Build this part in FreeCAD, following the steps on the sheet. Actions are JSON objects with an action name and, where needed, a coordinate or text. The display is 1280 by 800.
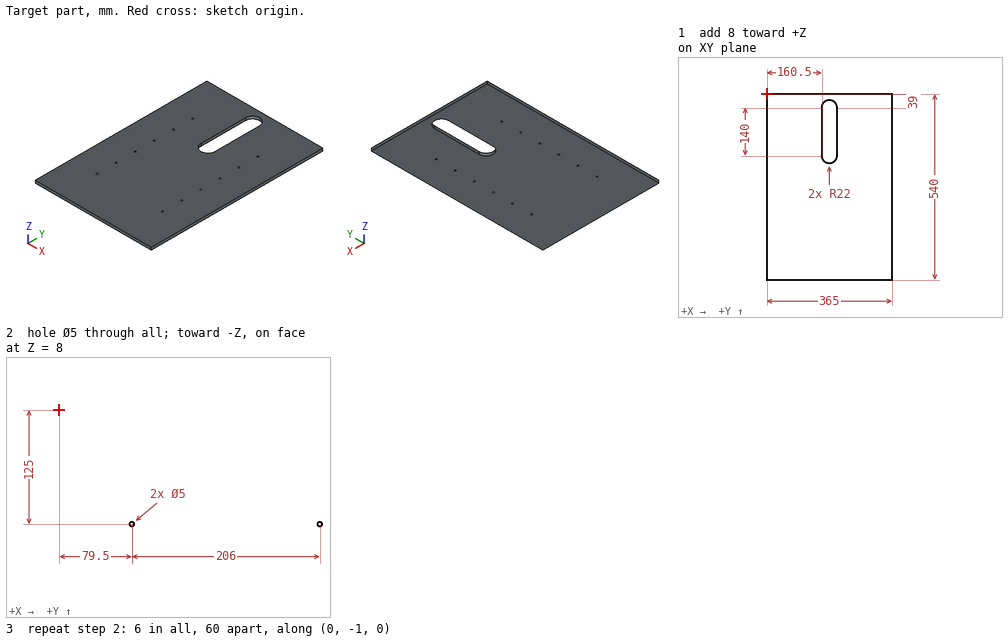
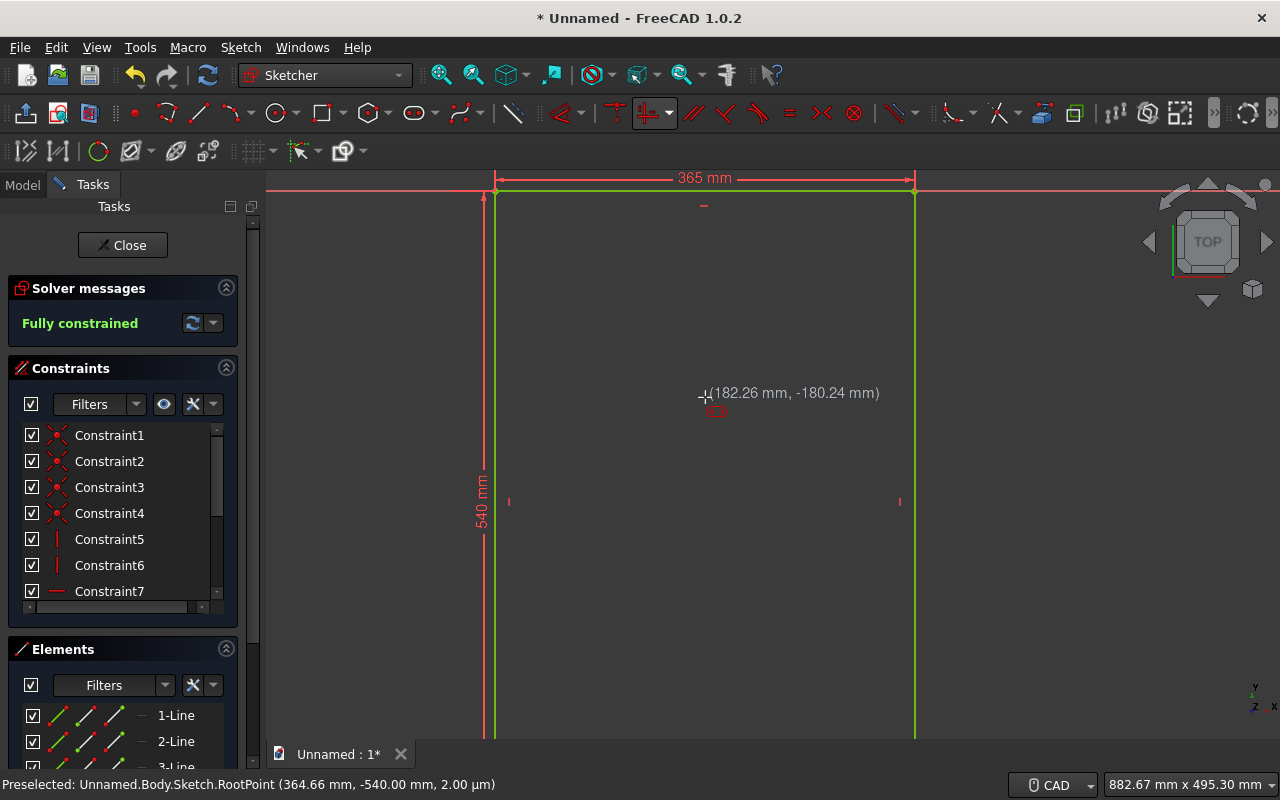
{"action": "left_click", "coordinate": [705, 397]}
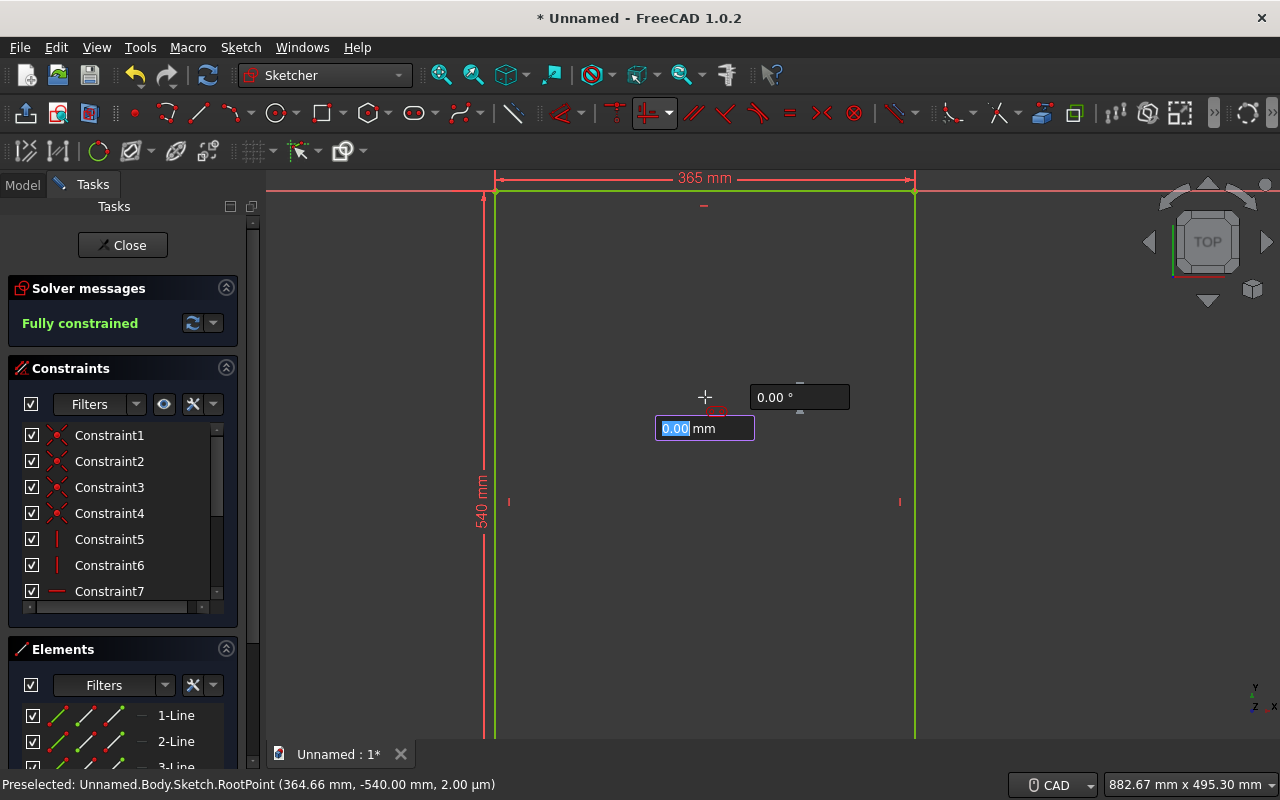
{"action": "left_click", "coordinate": [705, 236]}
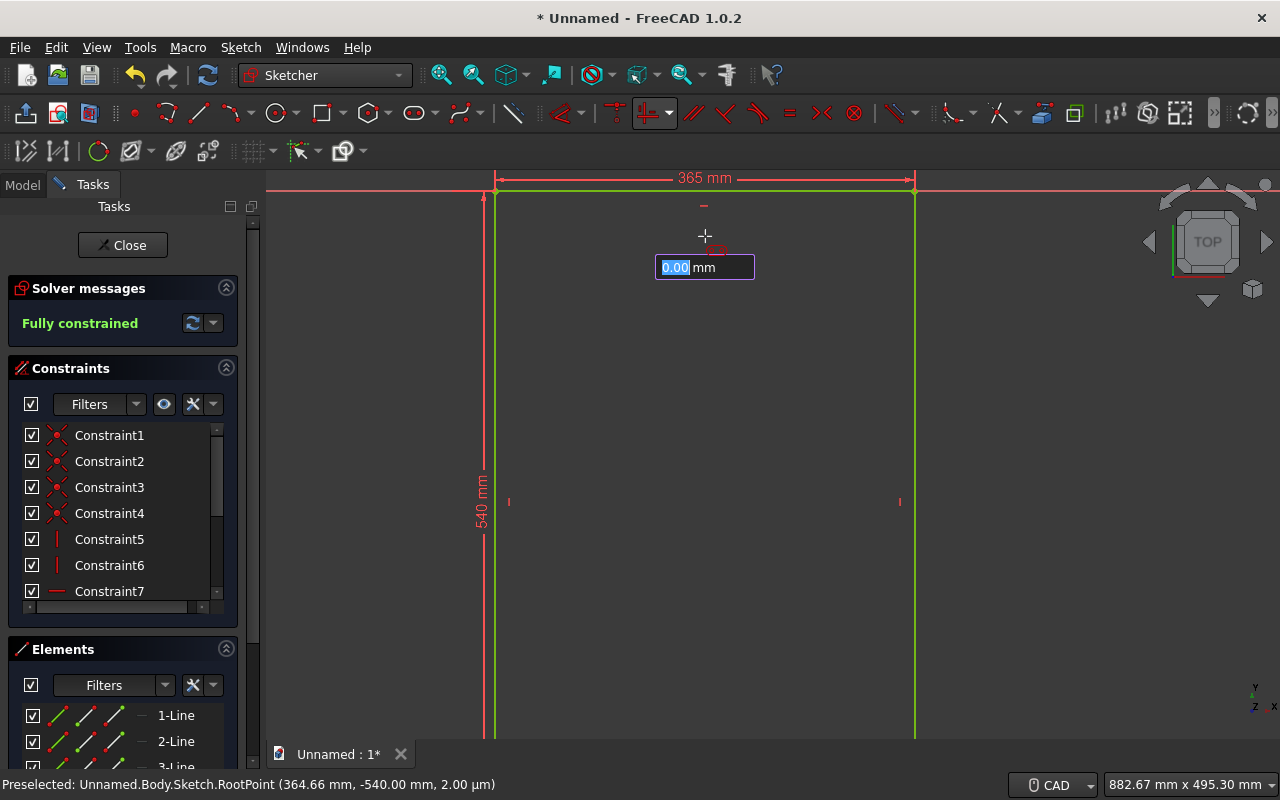
{"action": "left_click", "coordinate": [730, 317]}
{"action": "key", "text": "Escape"}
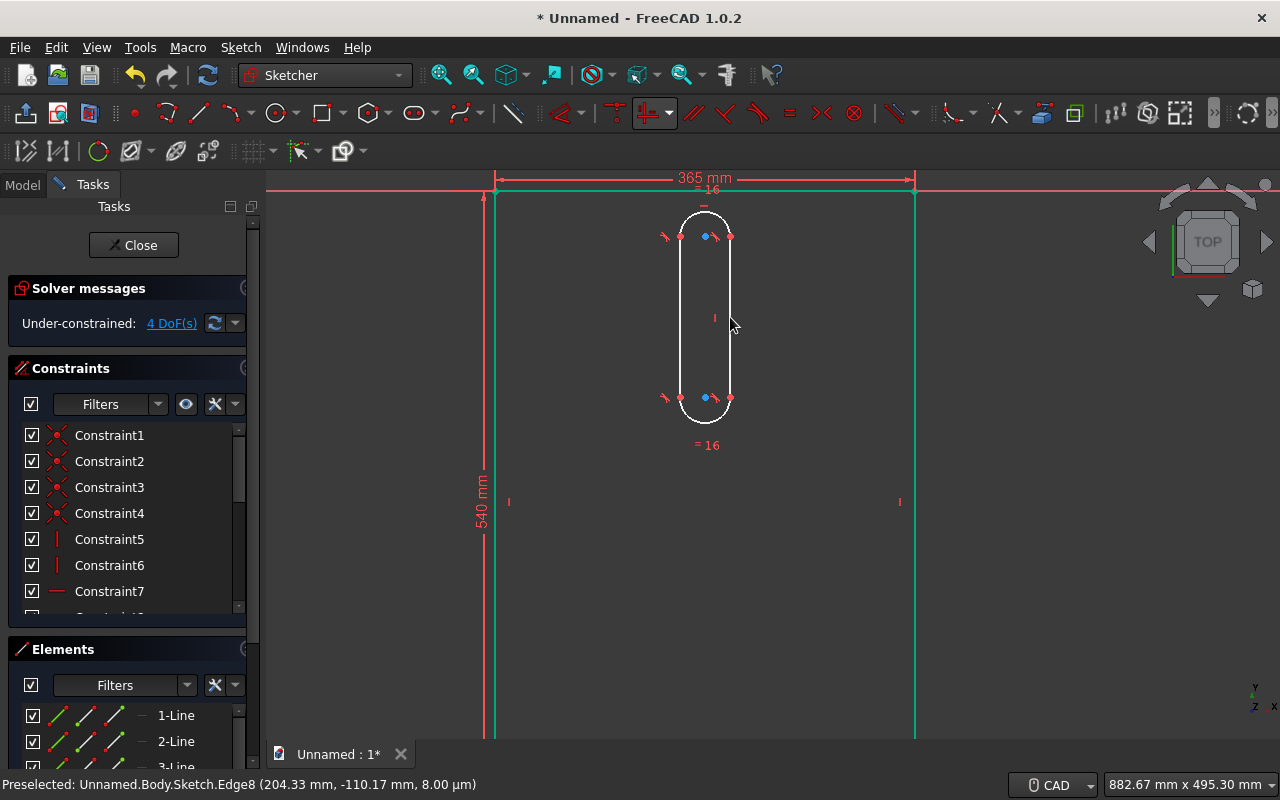
{"action": "left_click", "coordinate": [560, 114]}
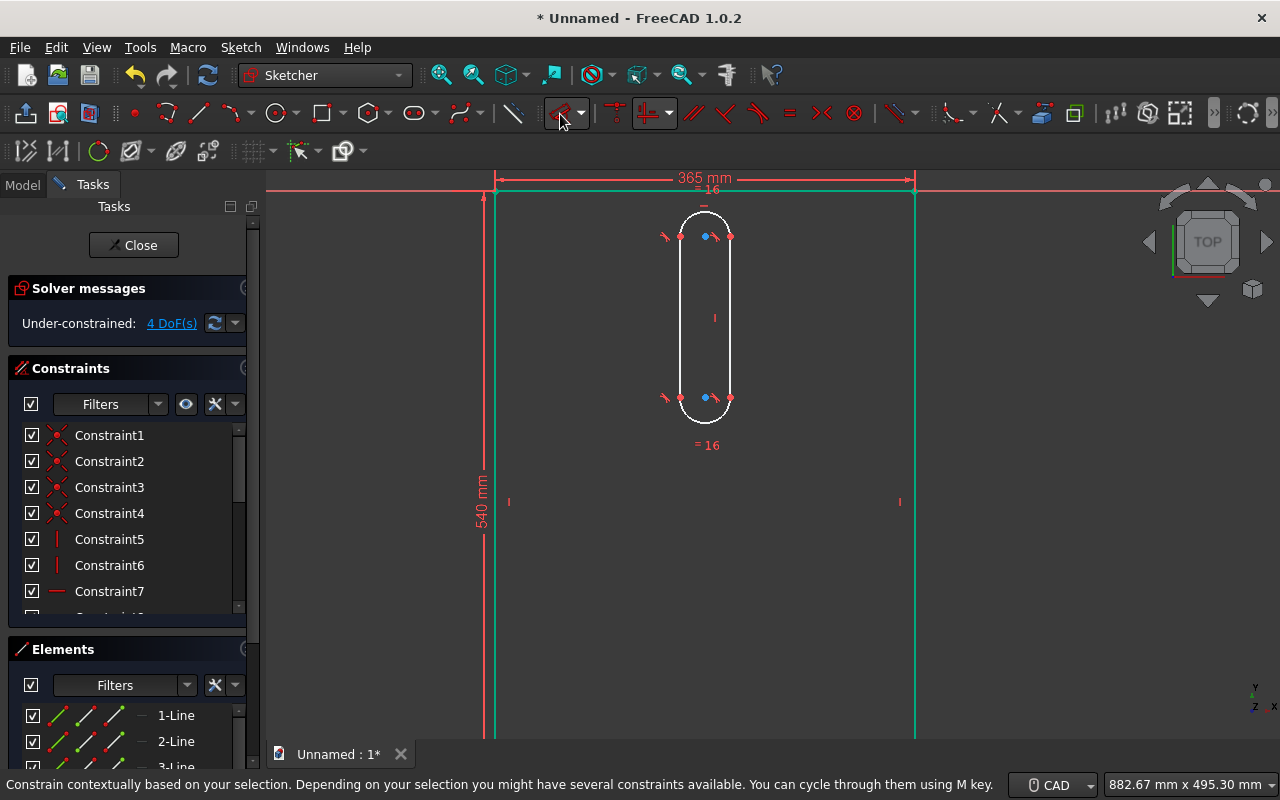
{"action": "scroll", "coordinate": [690, 418], "scroll_direction": "up", "scroll_amount": 3}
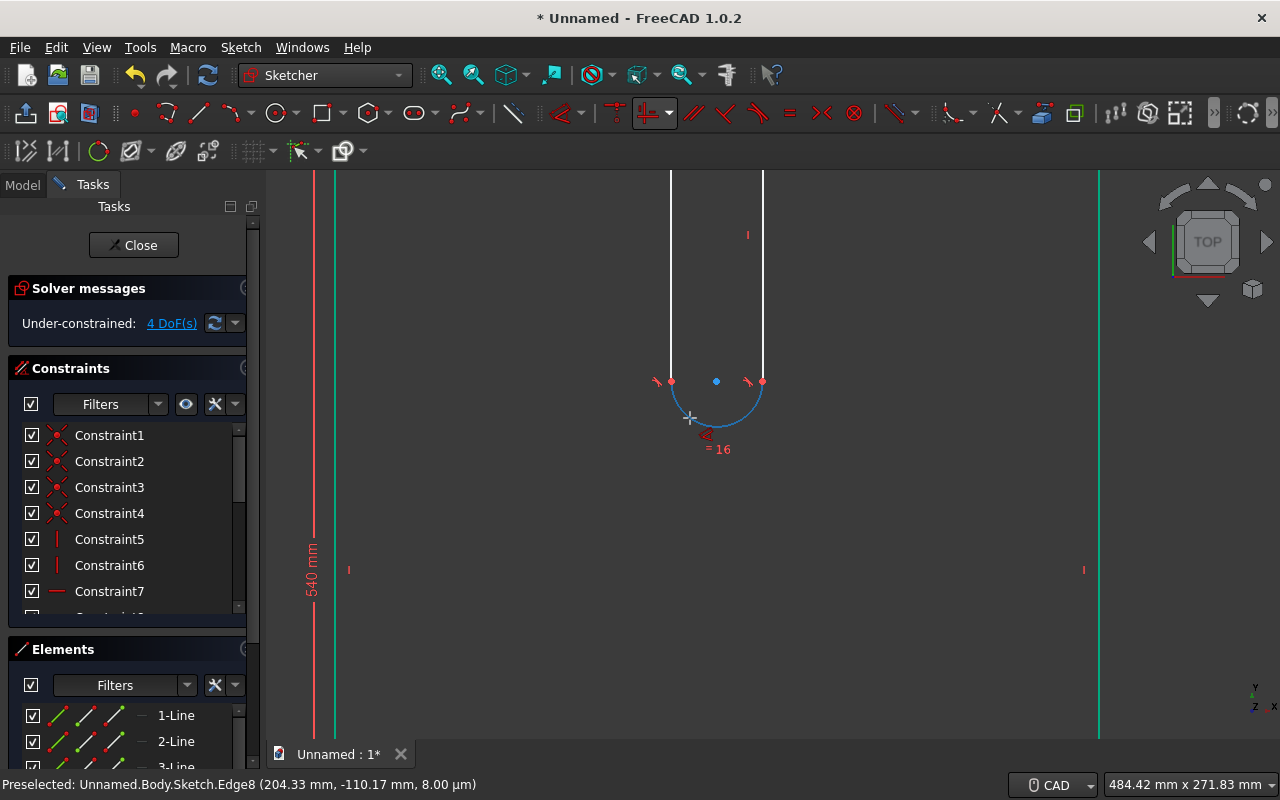
{"action": "left_click", "coordinate": [690, 418]}
{"action": "left_click", "coordinate": [671, 444]}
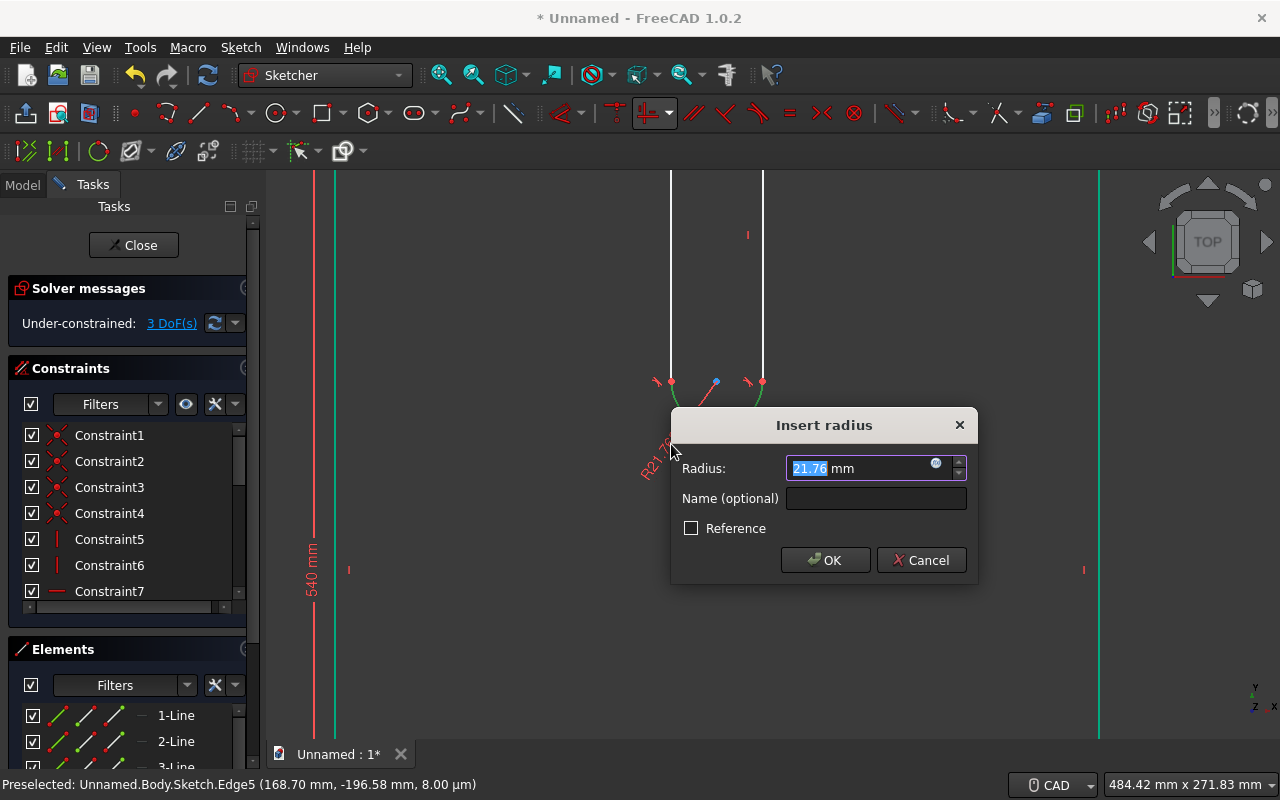
{"action": "type", "text": "22"}
{"action": "key", "text": "Return"}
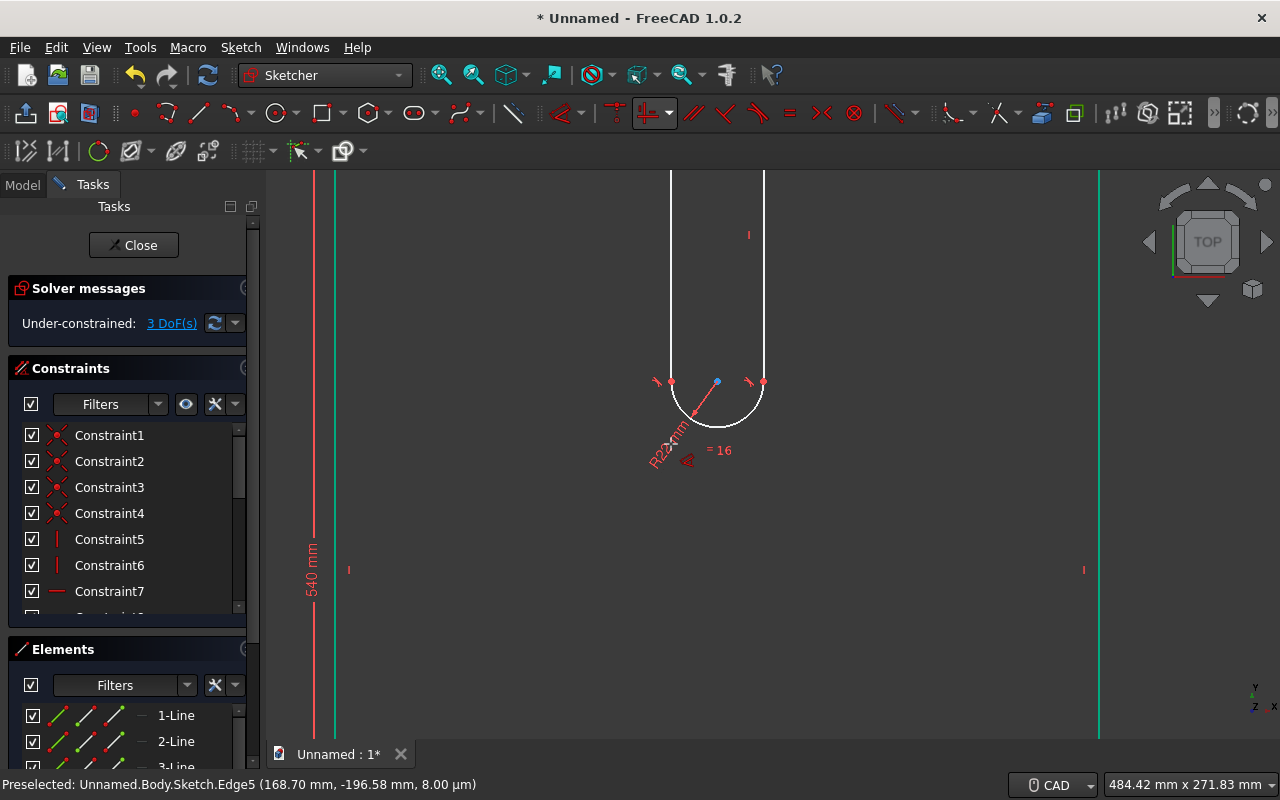
{"action": "left_click", "coordinate": [671, 293]}
{"action": "left_click", "coordinate": [637, 290]}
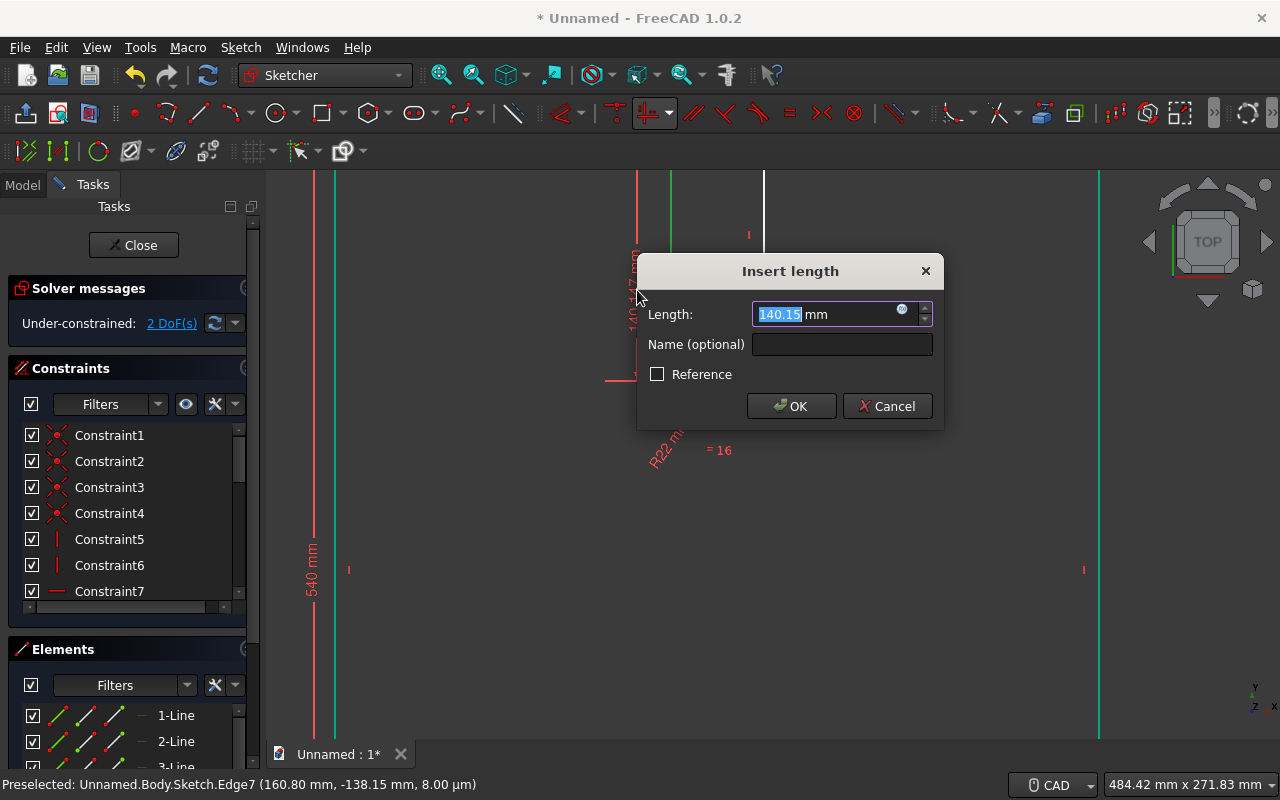
{"action": "type", "text": "140"}
{"action": "key", "text": "Return"}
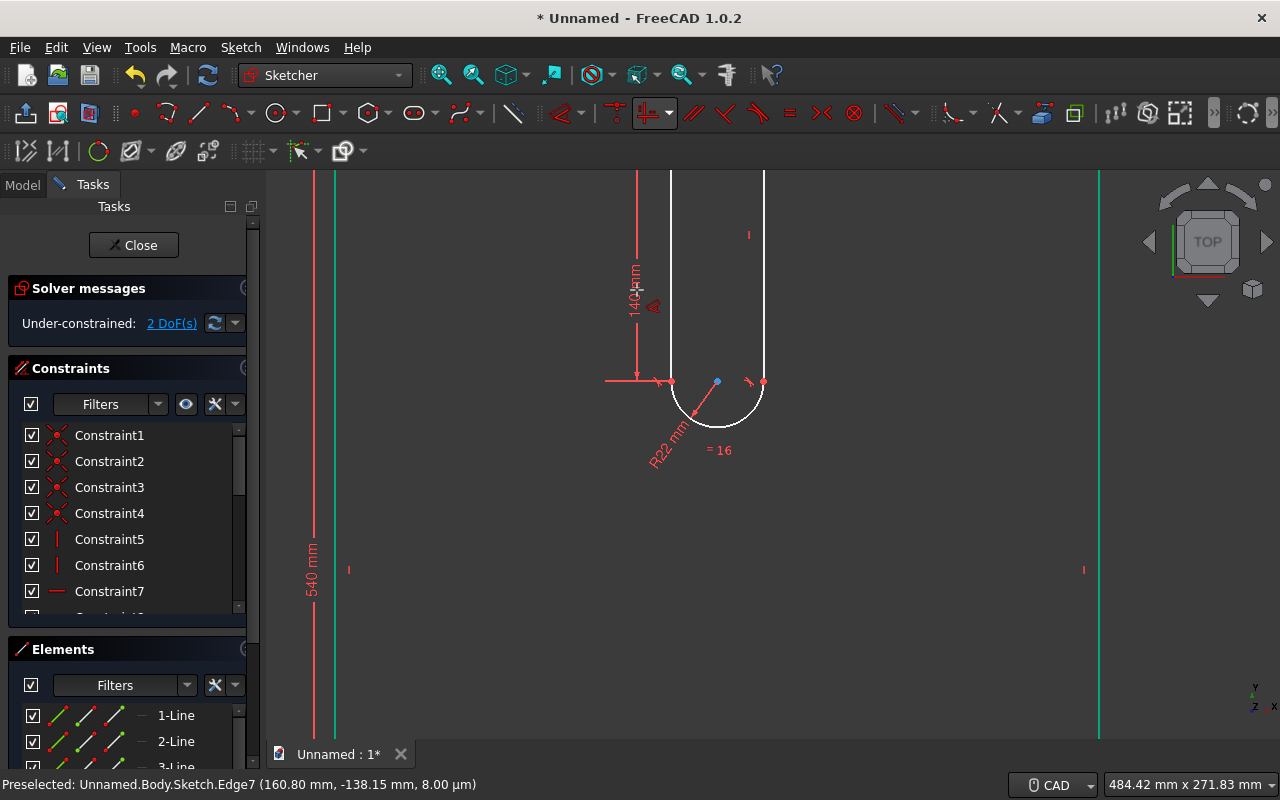
{"action": "scroll", "coordinate": [699, 405], "scroll_direction": "down", "scroll_amount": 6}